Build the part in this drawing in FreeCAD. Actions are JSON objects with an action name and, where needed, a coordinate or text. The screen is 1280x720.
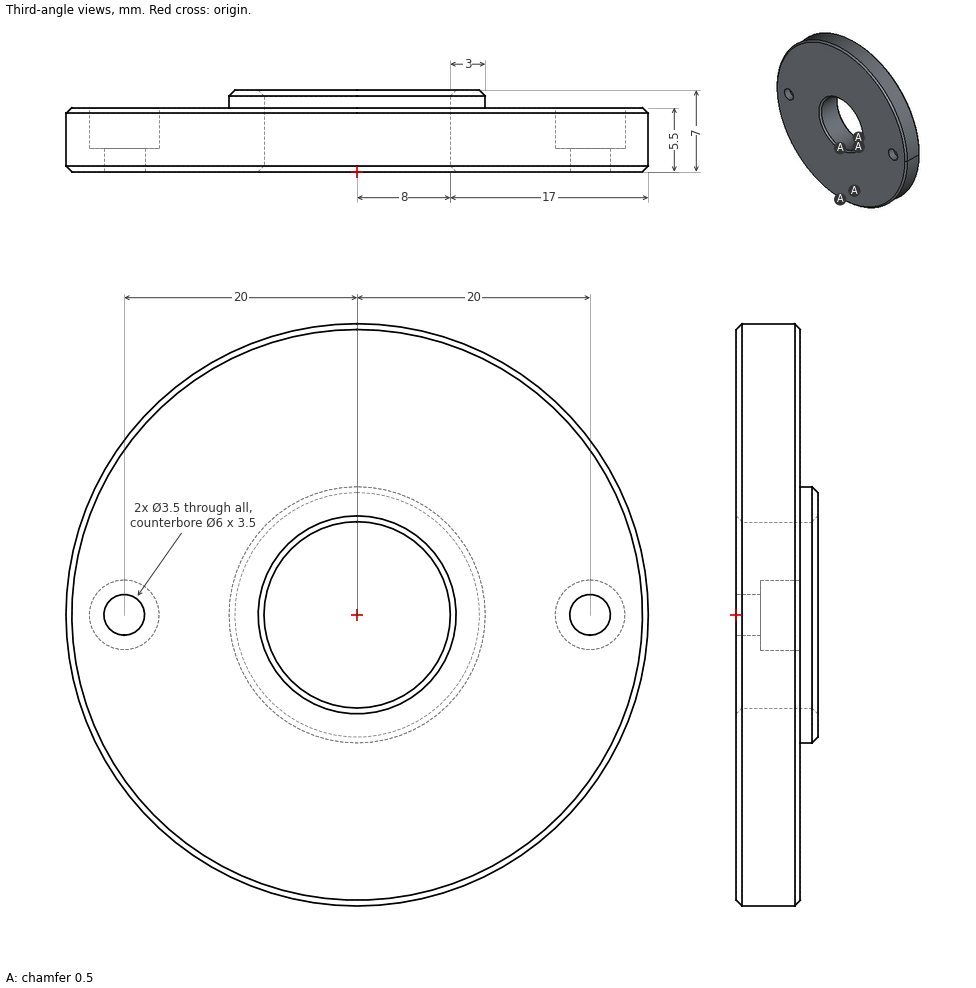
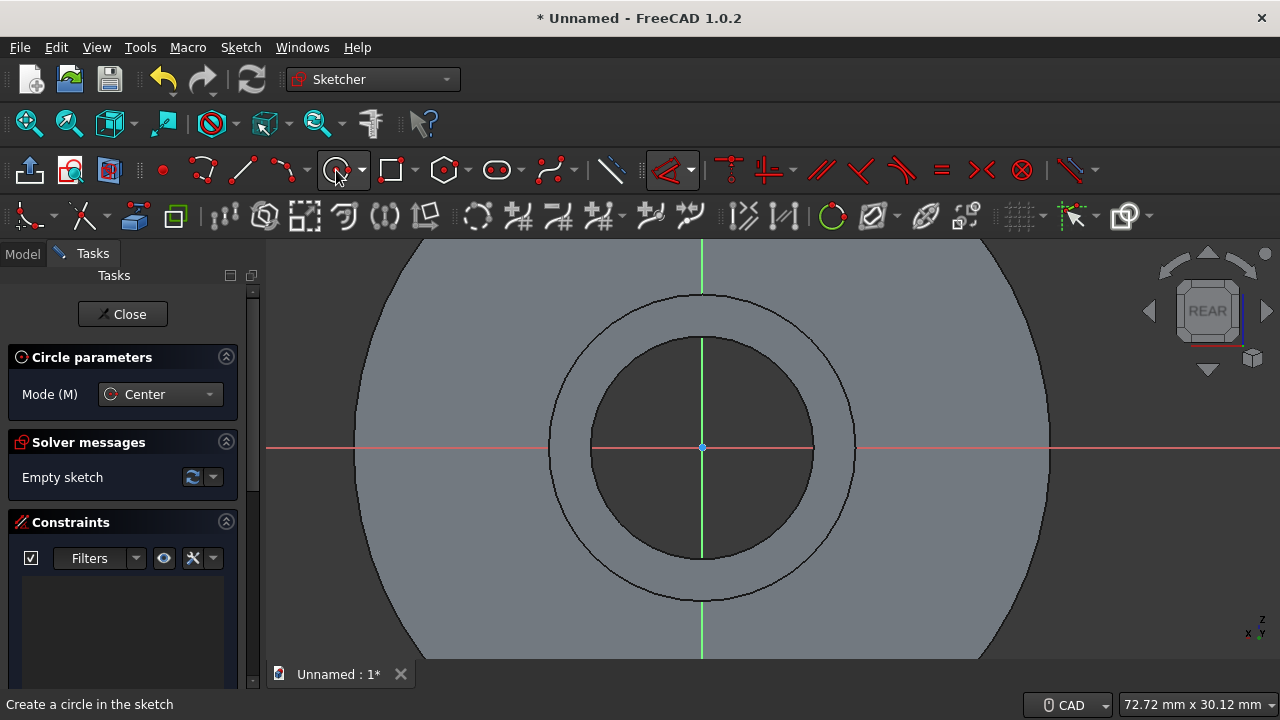
{"action": "left_click", "coordinate": [981, 448]}
{"action": "mouse_move", "coordinate": [998, 431]}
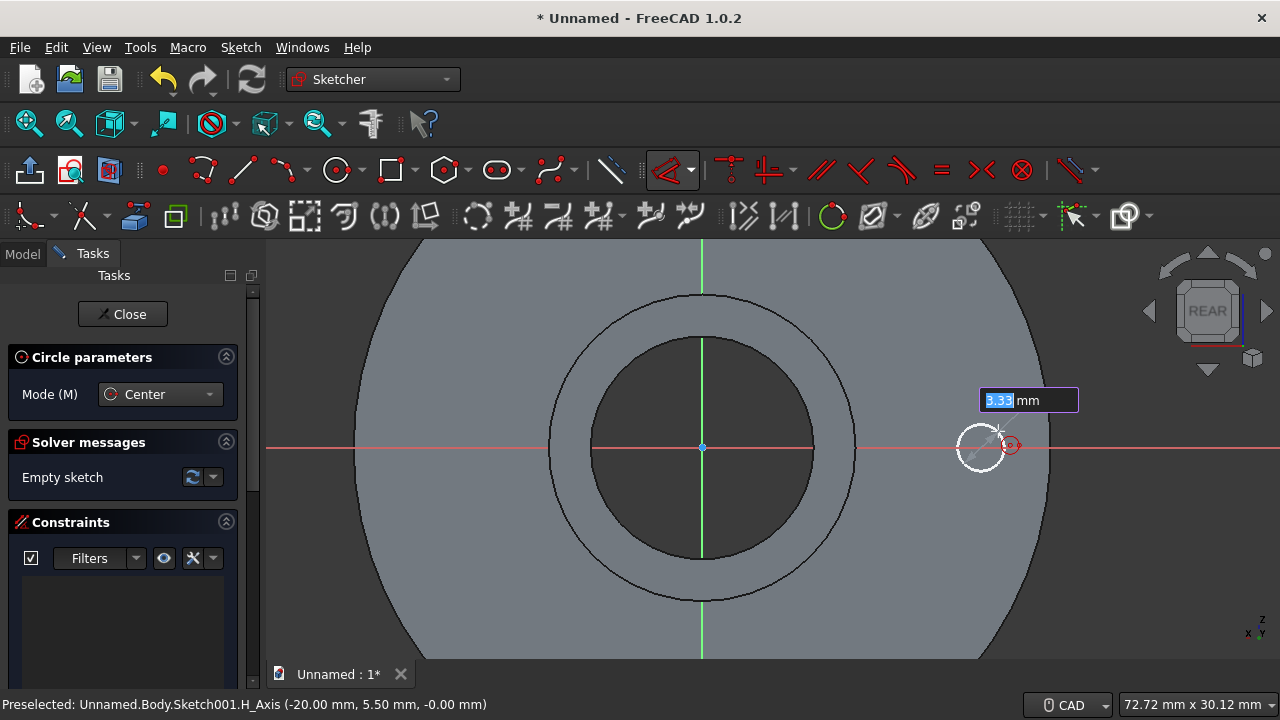
{"action": "type", "text": "3.5"}
{"action": "key", "text": "Return"}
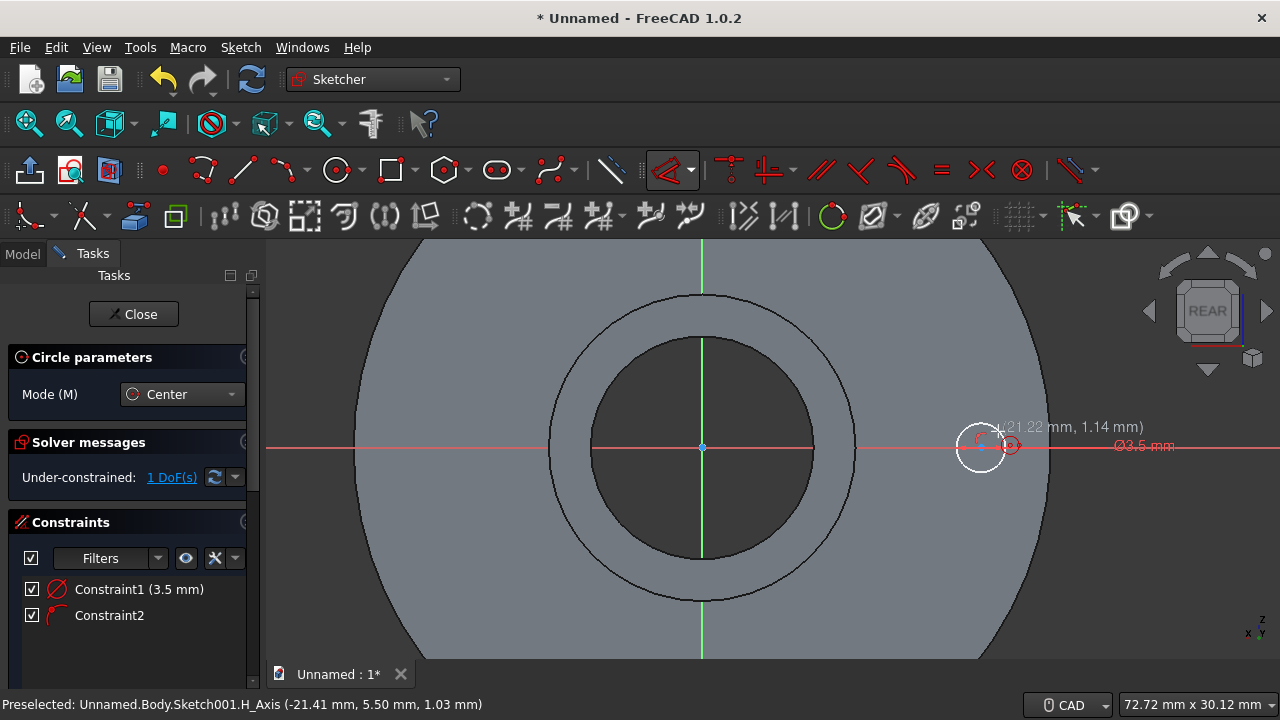
{"action": "left_click", "coordinate": [423, 448]}
{"action": "mouse_move", "coordinate": [441, 431]}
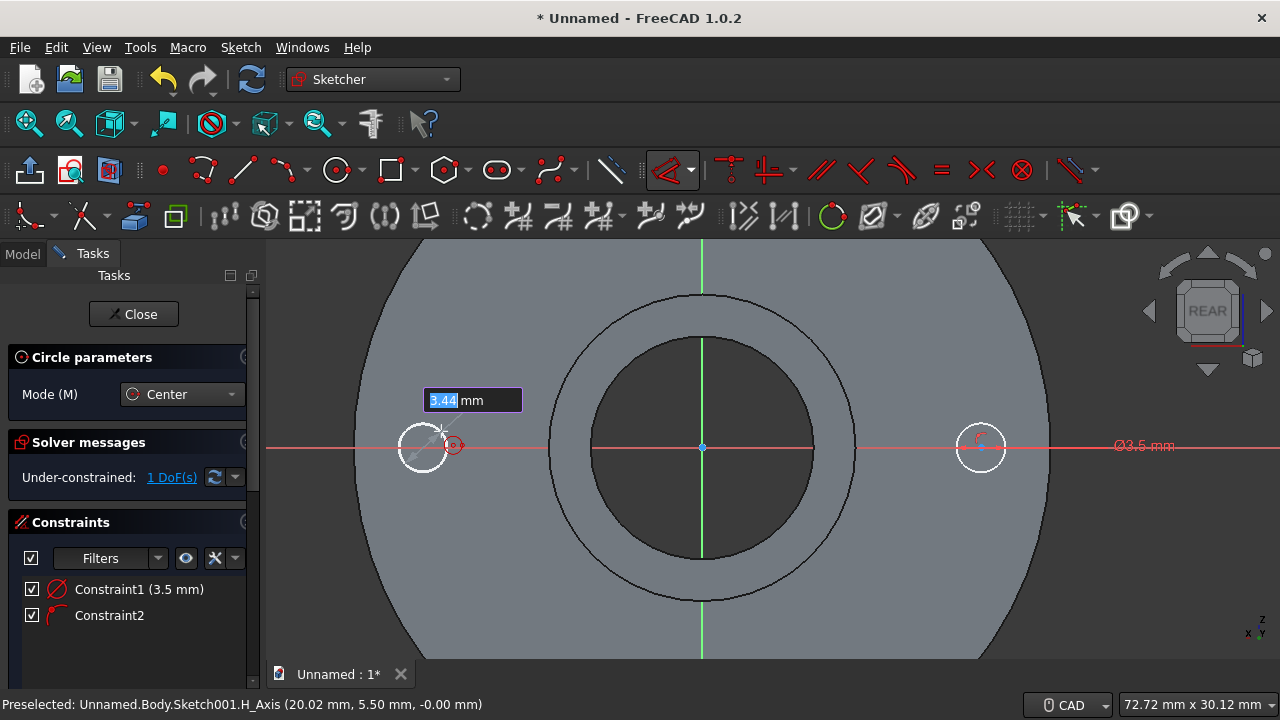
{"action": "type", "text": "3.5"}
{"action": "key", "text": "Return"}
{"action": "key", "text": "Escape"}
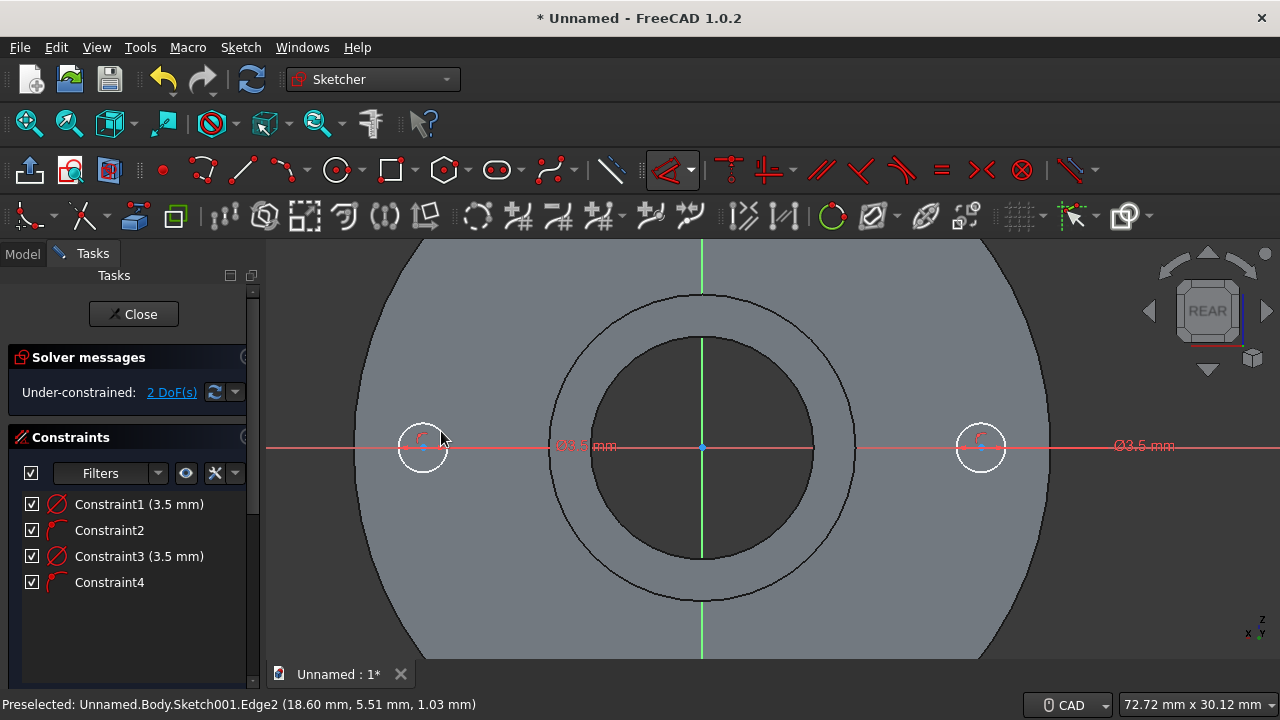
{"action": "left_click", "coordinate": [981, 448]}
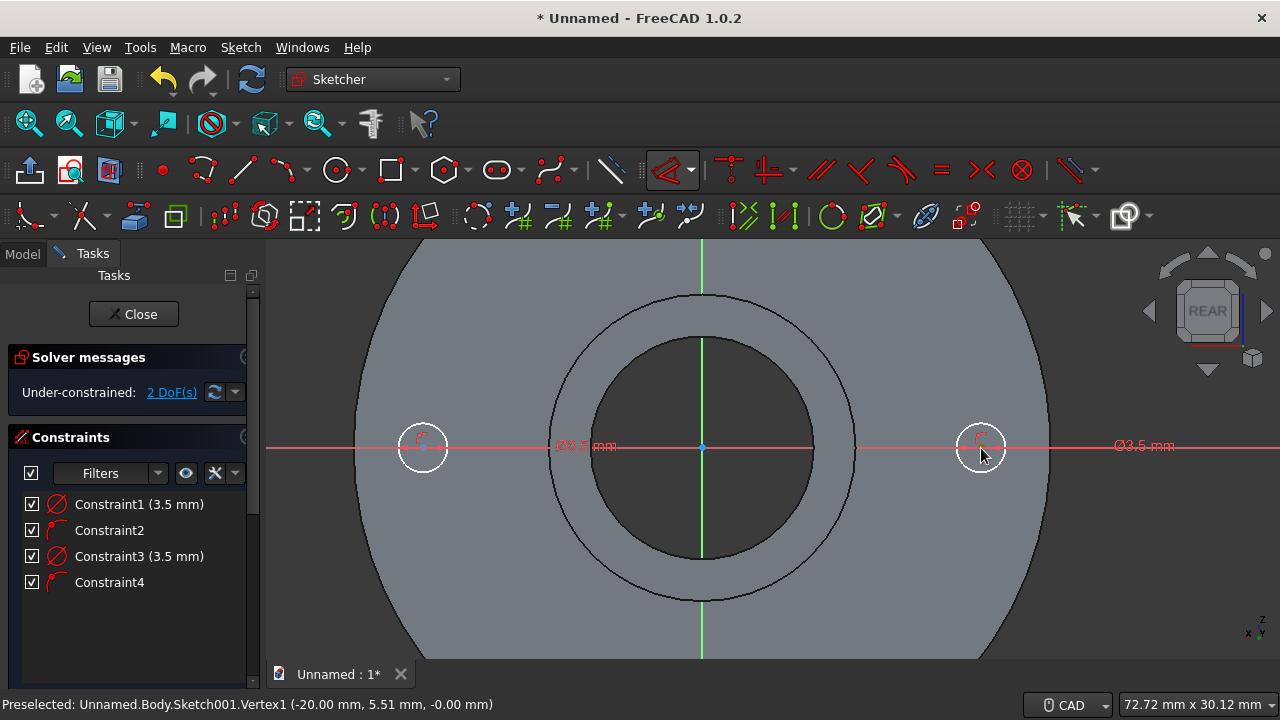
{"action": "key", "text": "l"}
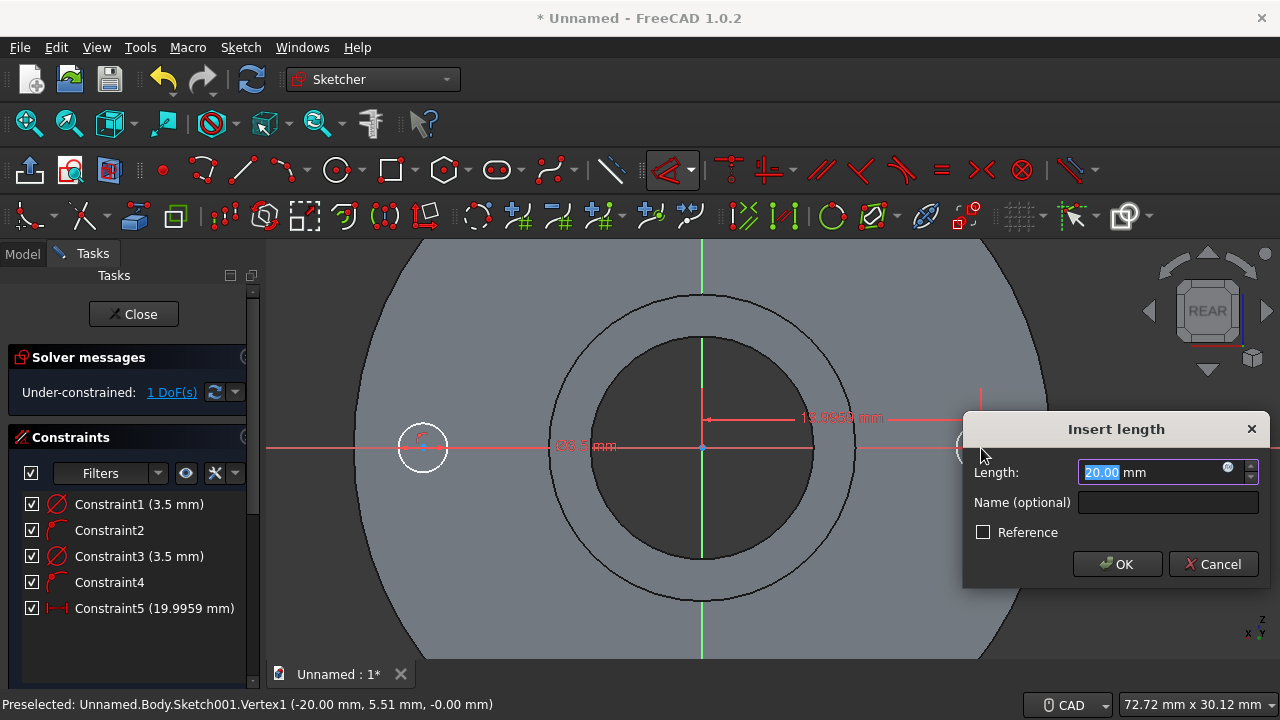
{"action": "type", "text": "20"}
{"action": "key", "text": "Return"}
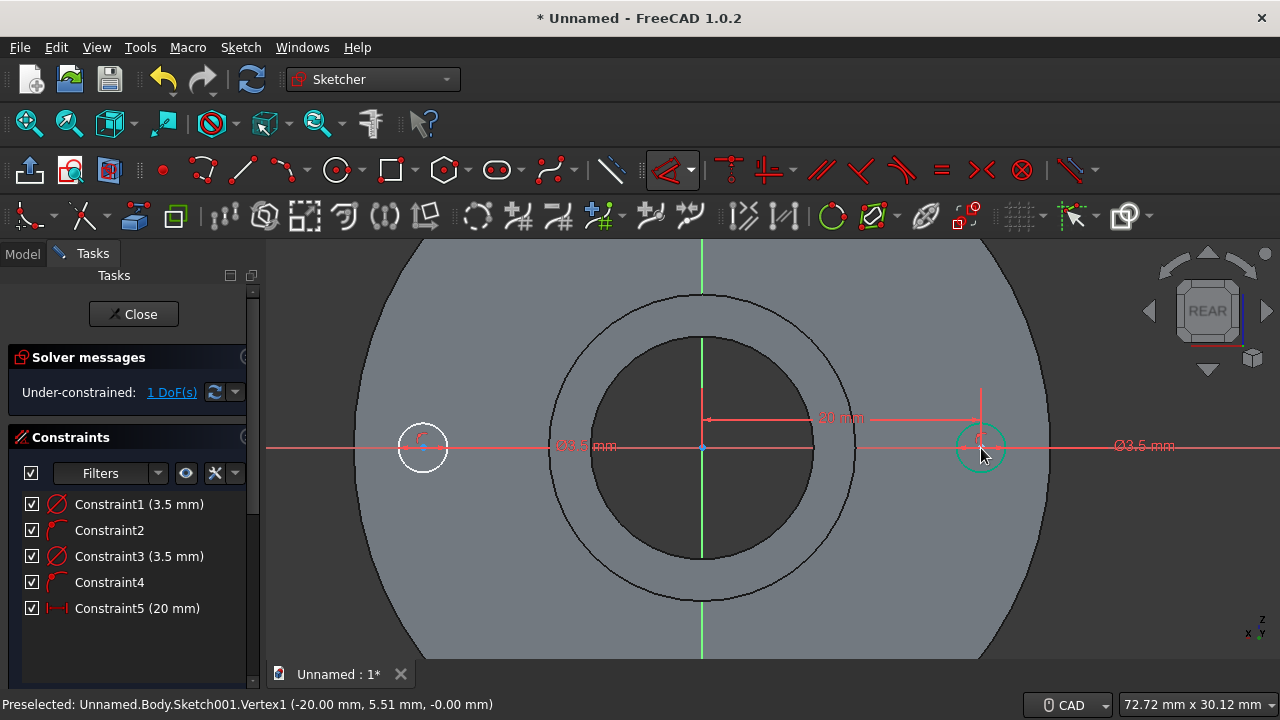
{"action": "left_click", "coordinate": [423, 448]}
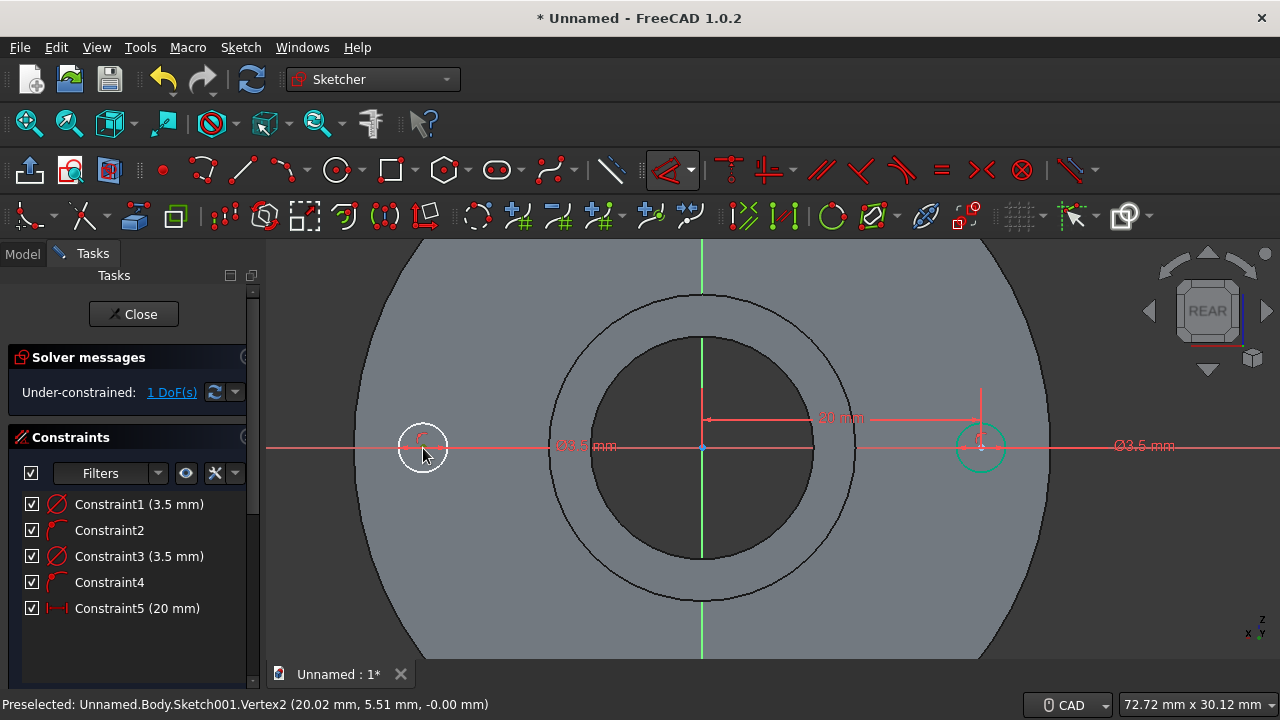
{"action": "left_click", "coordinate": [694, 170]}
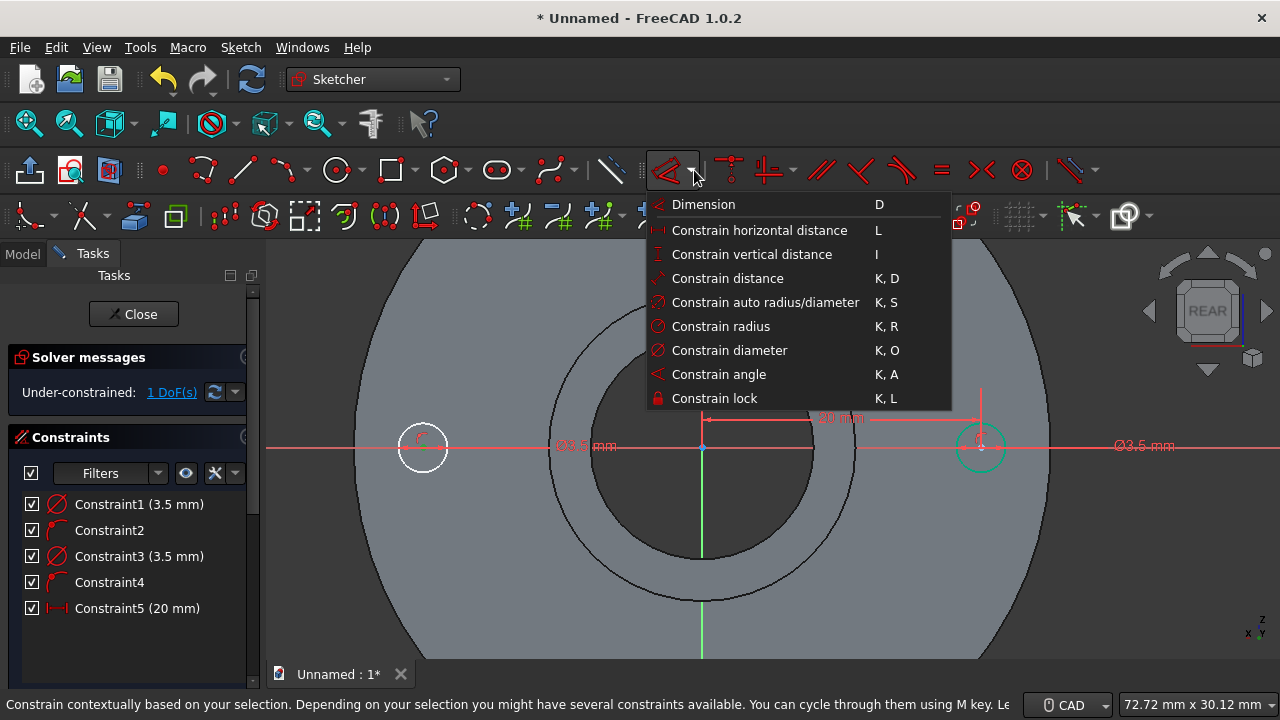
{"action": "left_click", "coordinate": [799, 230]}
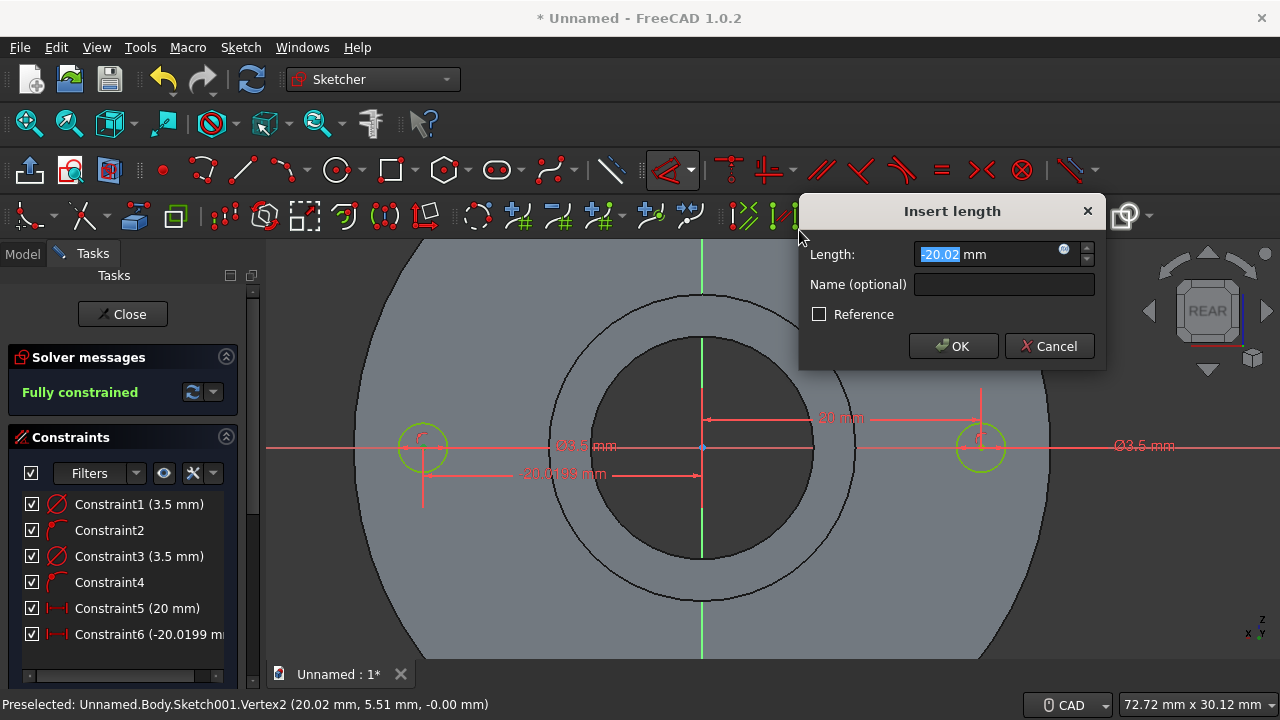
{"action": "type", "text": "-20"}
{"action": "key", "text": "Return"}